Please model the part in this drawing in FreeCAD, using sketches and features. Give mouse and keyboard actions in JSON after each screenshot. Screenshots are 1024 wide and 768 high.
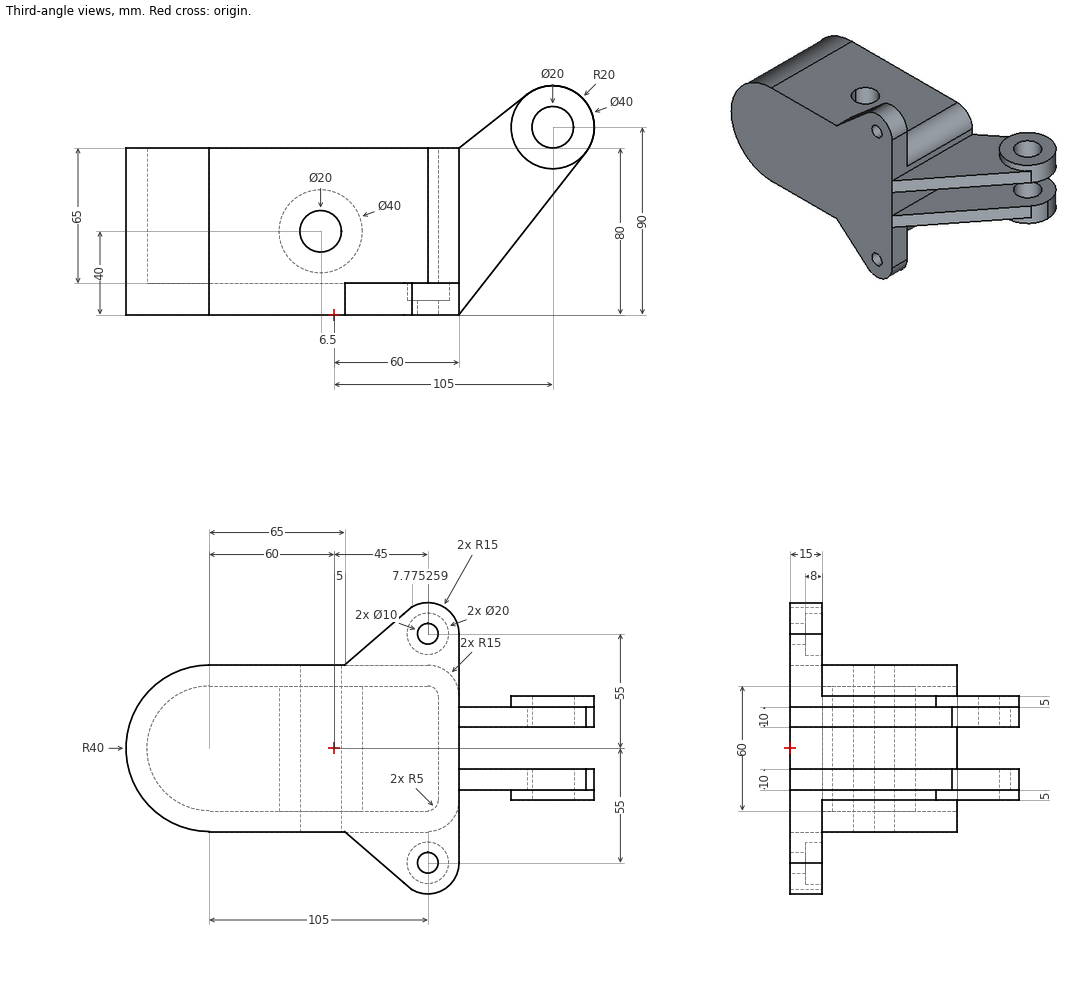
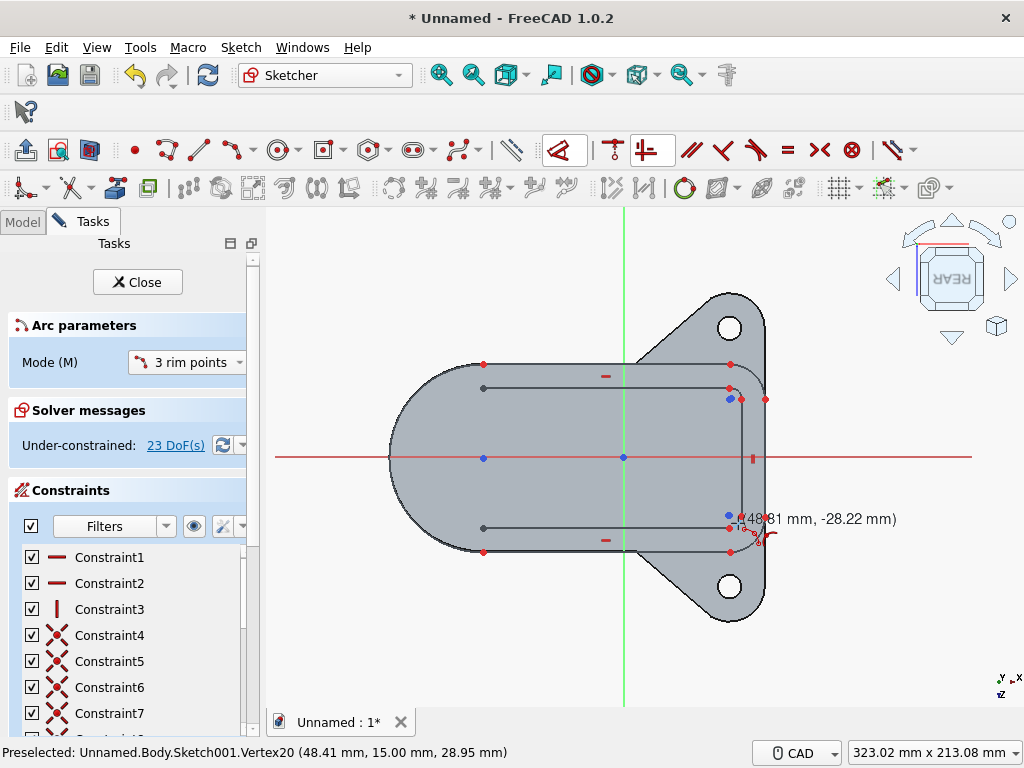
{"action": "left_click", "coordinate": [483, 528]}
{"action": "left_click", "coordinate": [483, 388]}
{"action": "left_click", "coordinate": [416, 436]}
{"action": "key", "text": "Escape"}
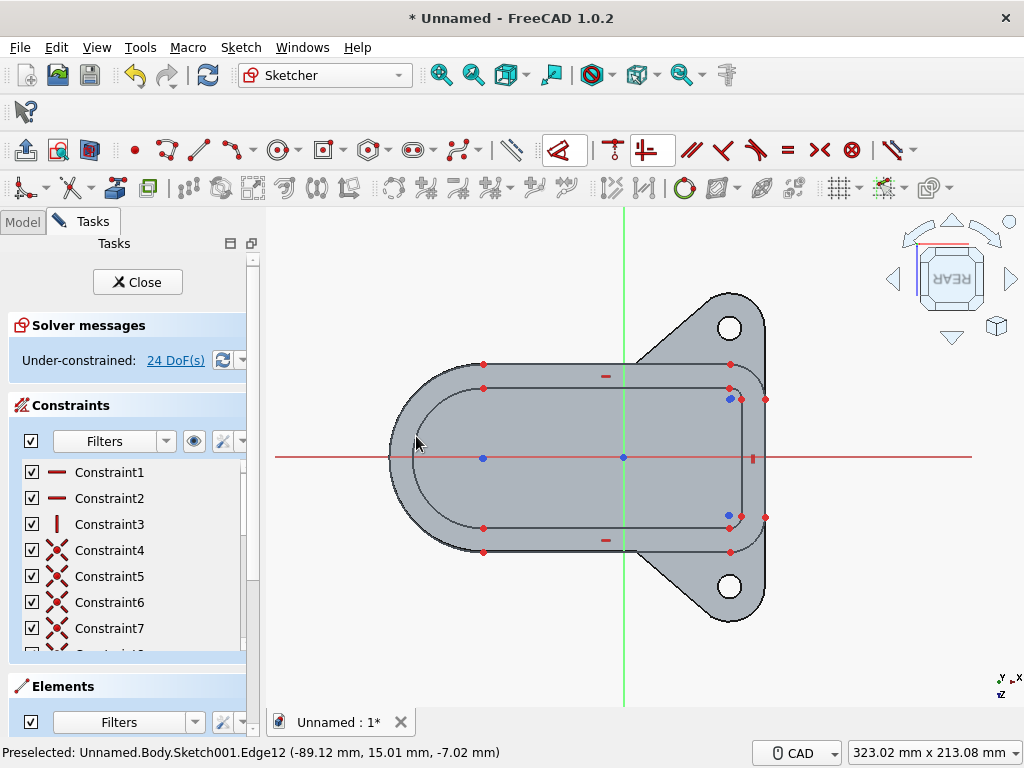
{"action": "left_click", "coordinate": [656, 364]}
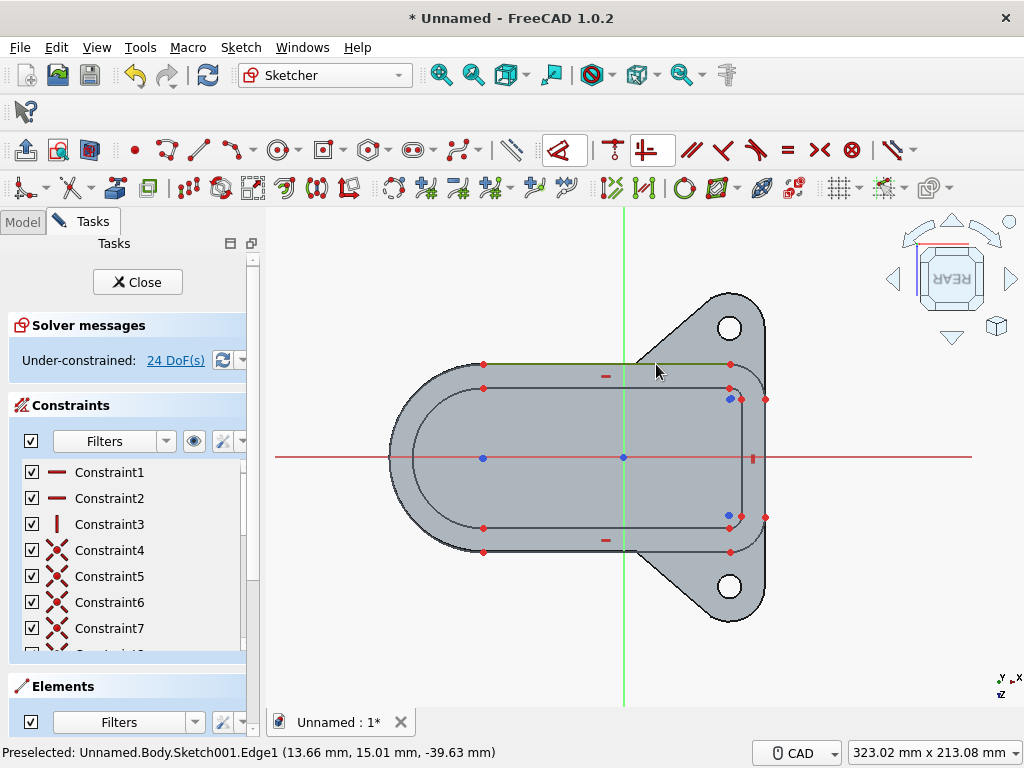
{"action": "left_click", "coordinate": [761, 384]}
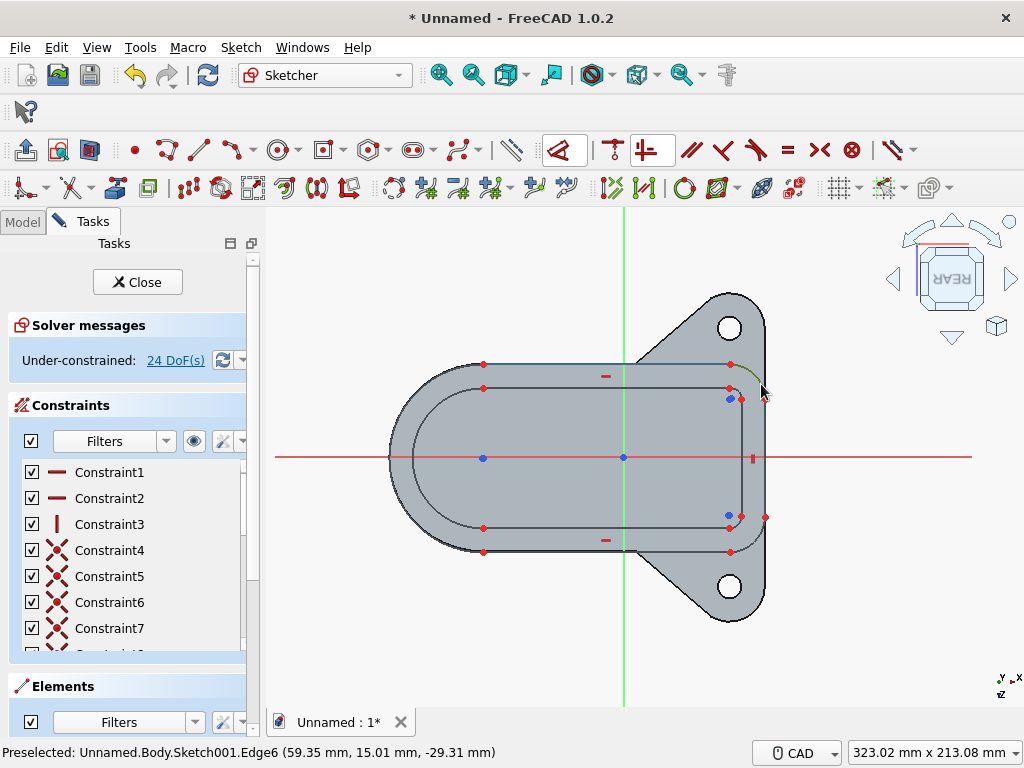
{"action": "left_click", "coordinate": [756, 150]}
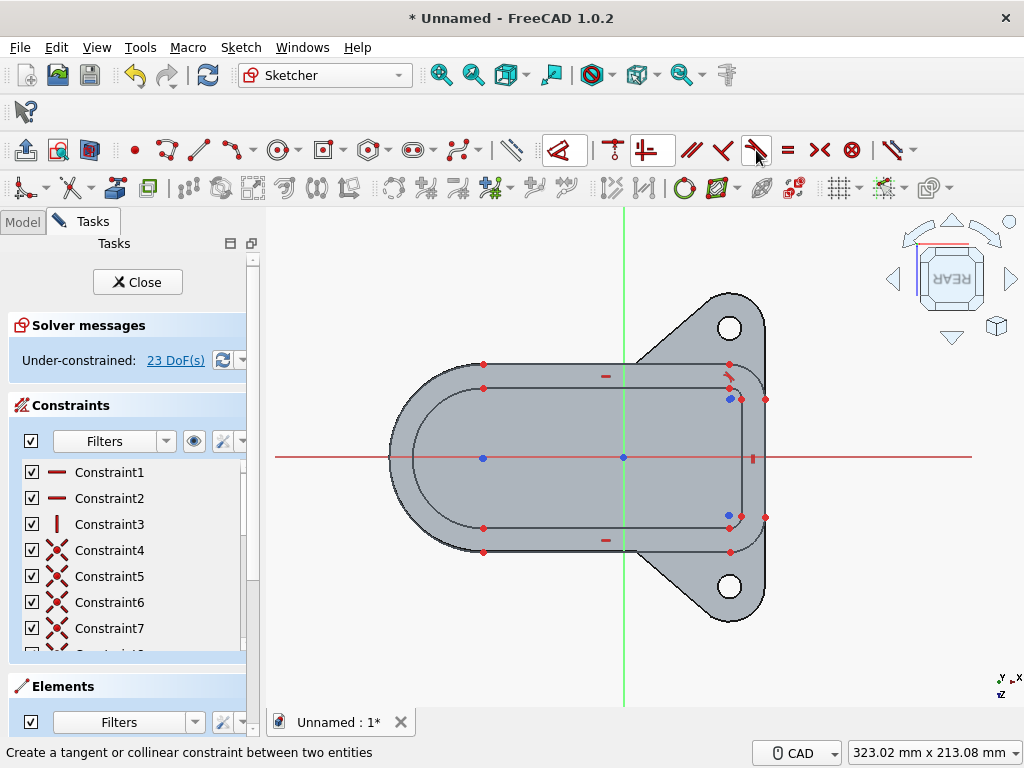
{"action": "left_click", "coordinate": [557, 552]}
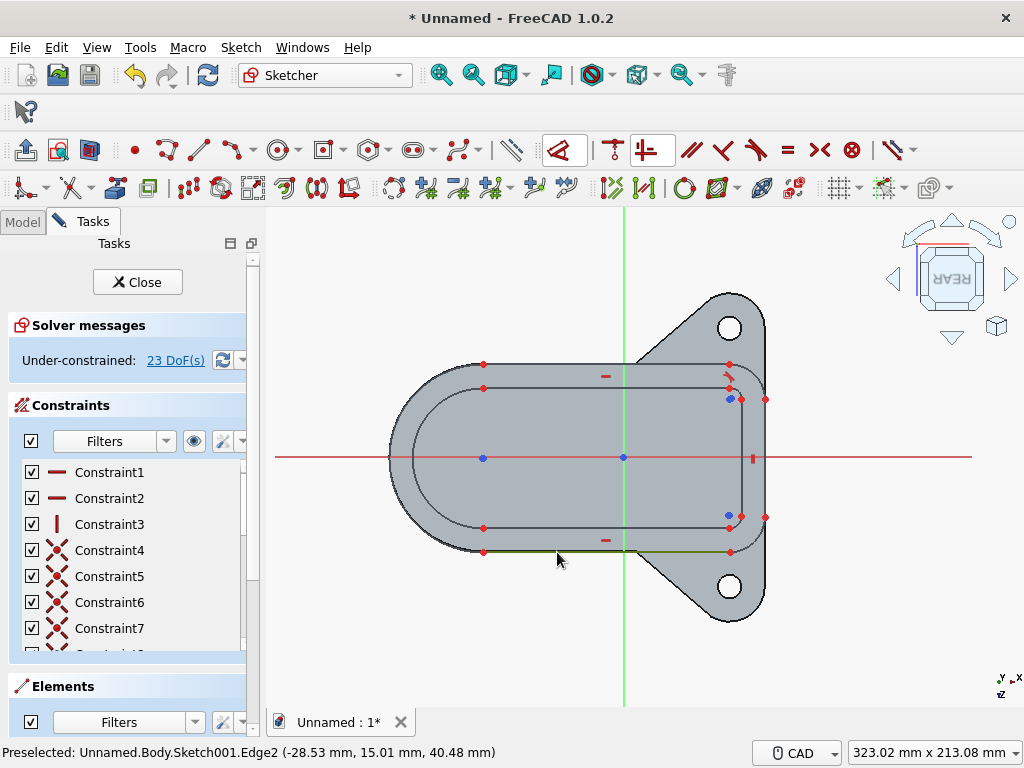
{"action": "left_click", "coordinate": [746, 548]}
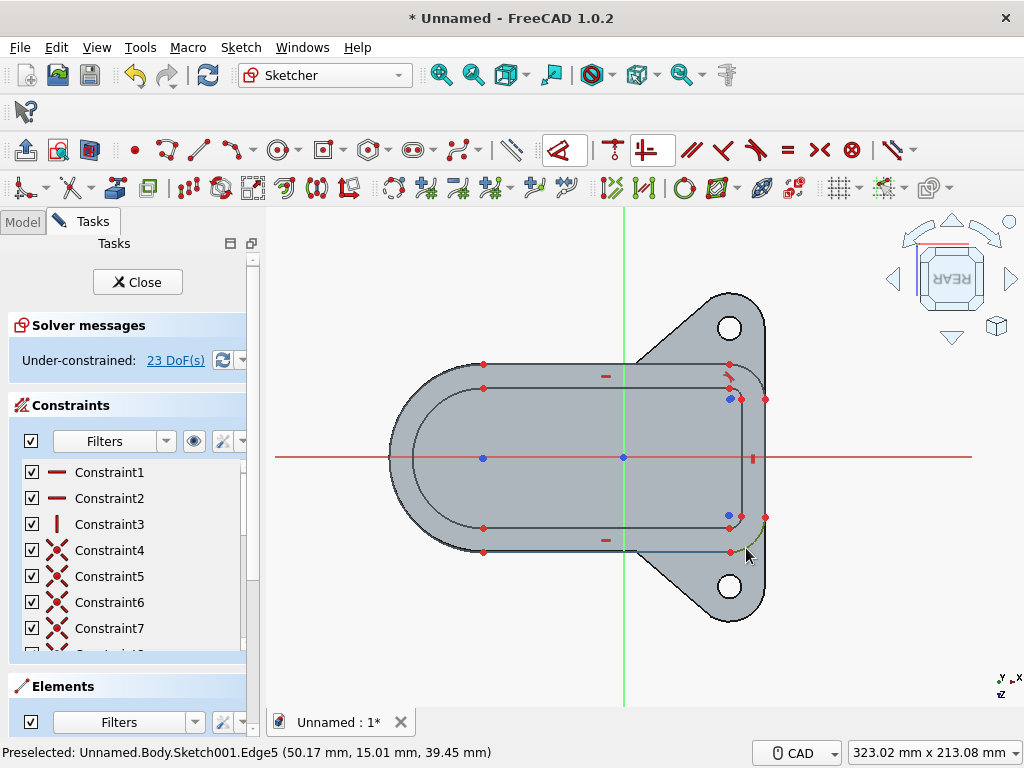
{"action": "left_click", "coordinate": [756, 150]}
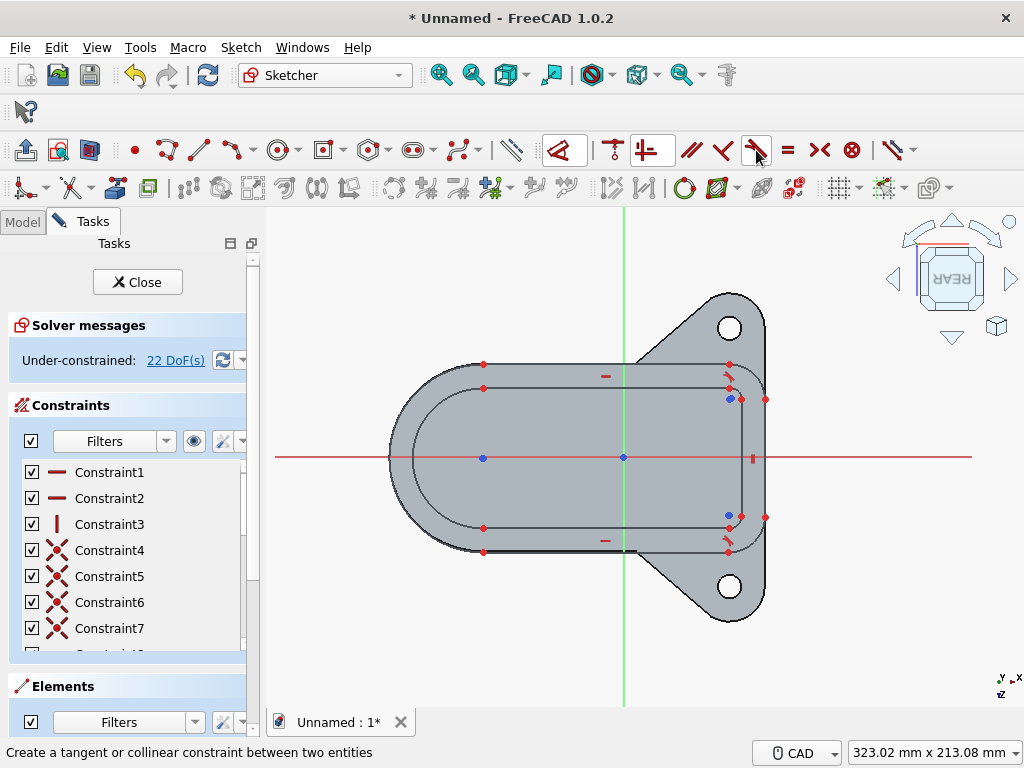
{"action": "left_click", "coordinate": [765, 482]}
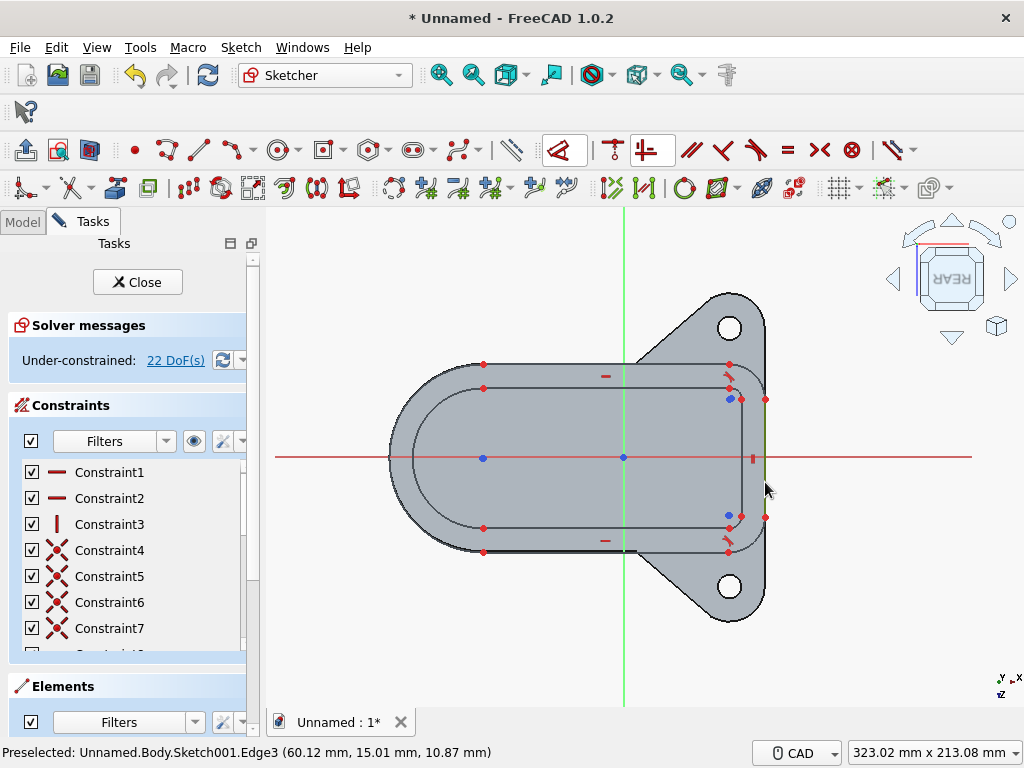
{"action": "left_click", "coordinate": [745, 549]}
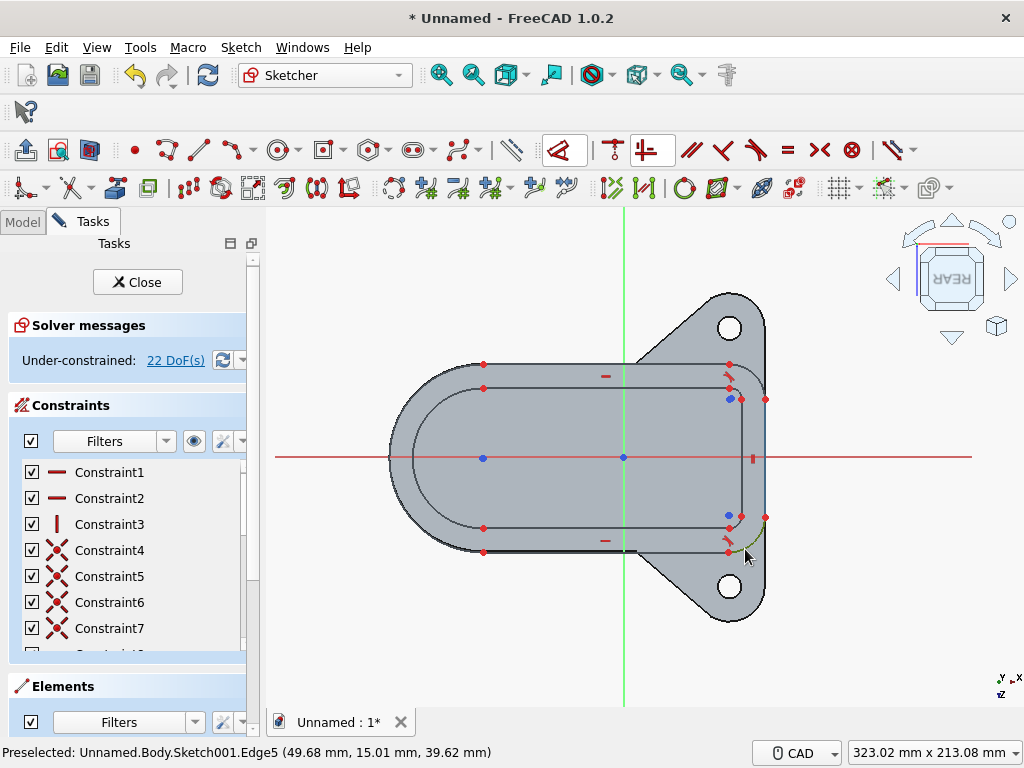
{"action": "left_click", "coordinate": [756, 150]}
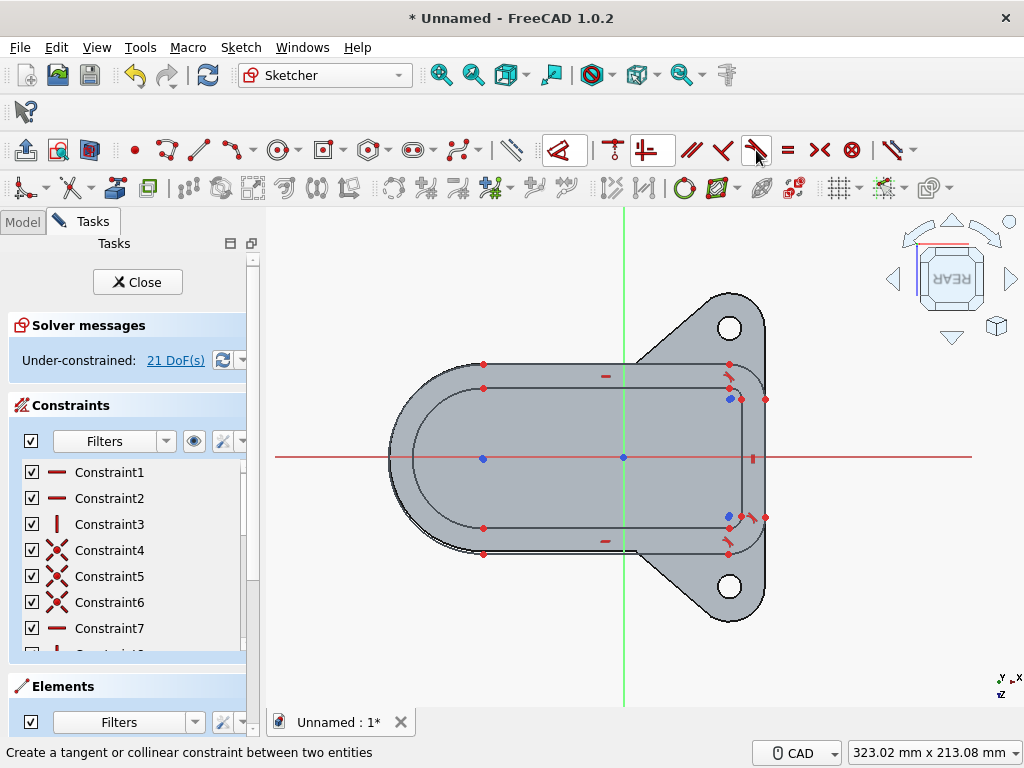
{"action": "left_click", "coordinate": [765, 482]}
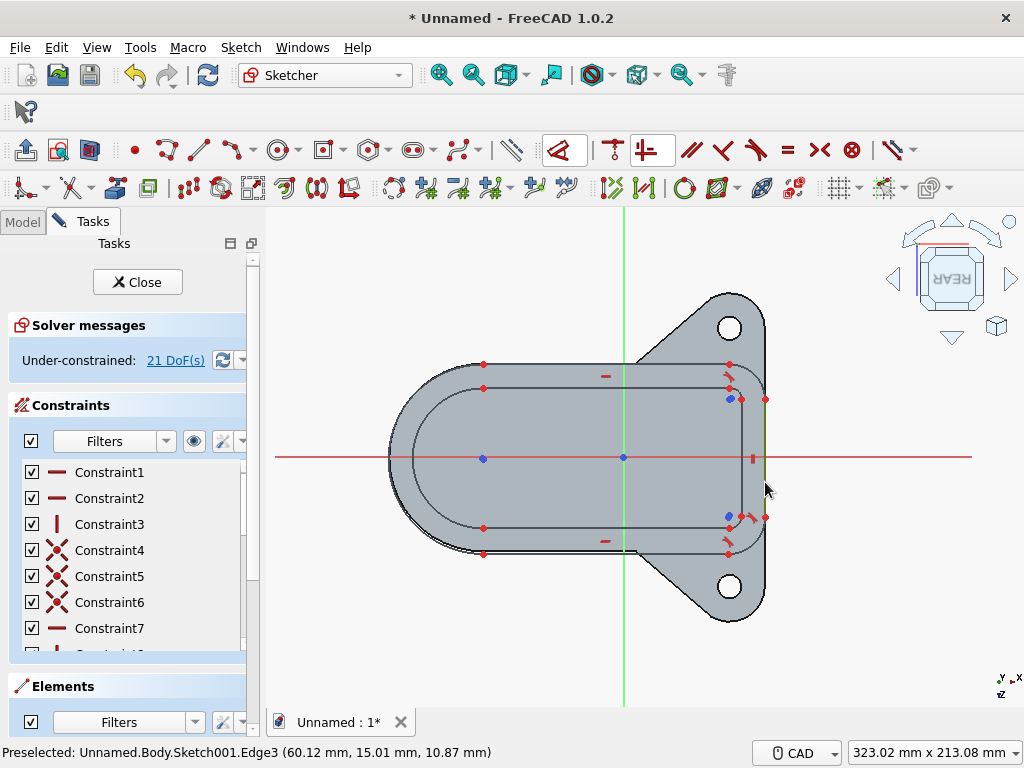
{"action": "left_click", "coordinate": [761, 384]}